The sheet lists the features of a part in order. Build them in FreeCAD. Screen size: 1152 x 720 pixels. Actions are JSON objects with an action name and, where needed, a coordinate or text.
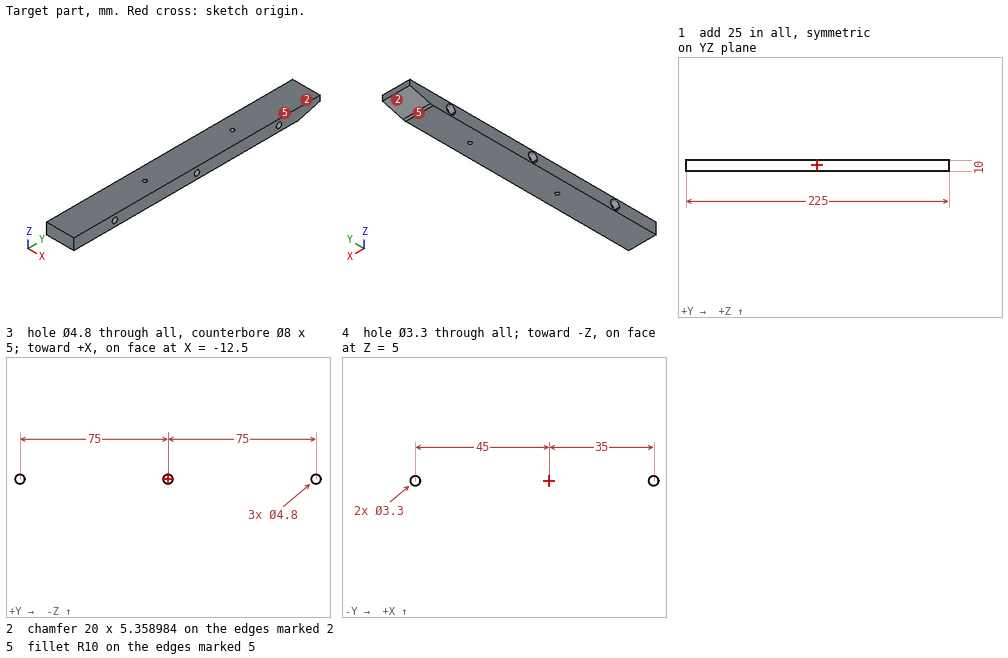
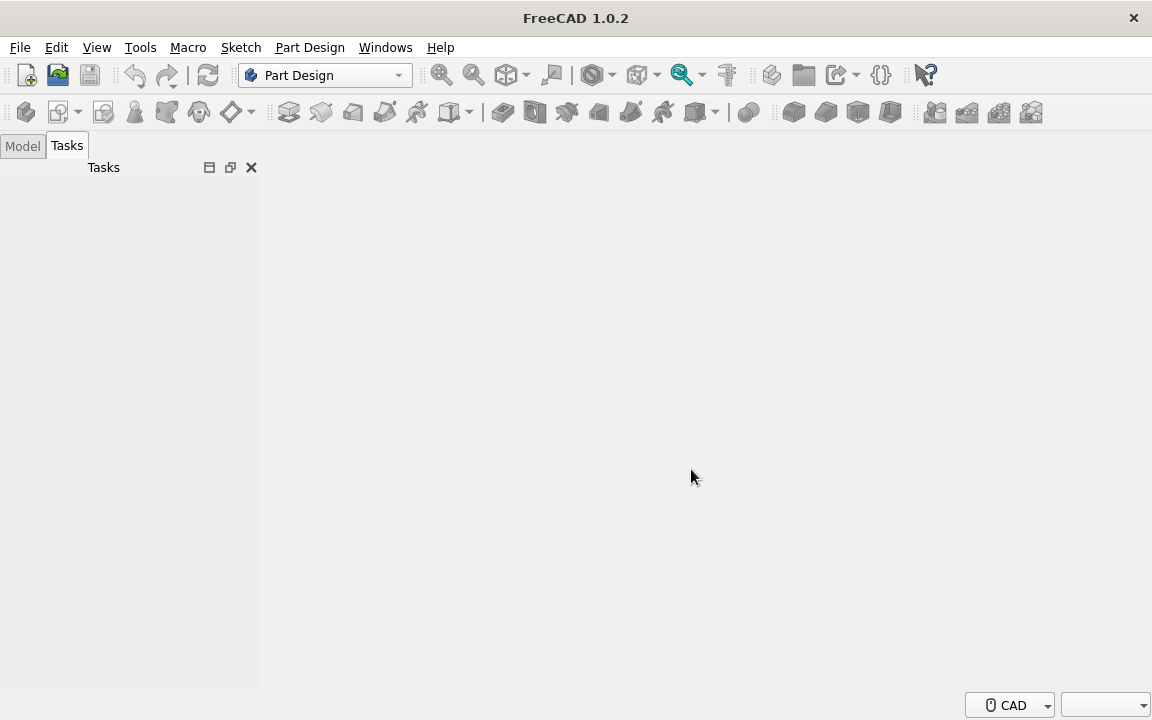
{"action": "key", "text": "ctrl+n"}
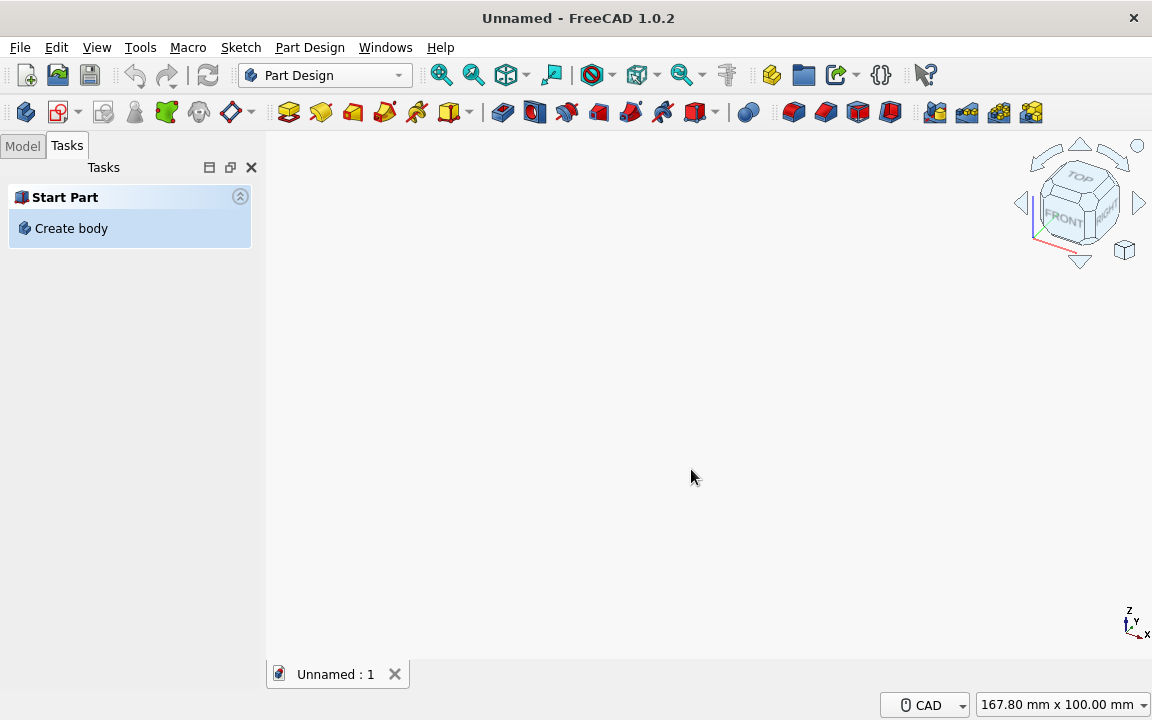
{"action": "left_click", "coordinate": [58, 112]}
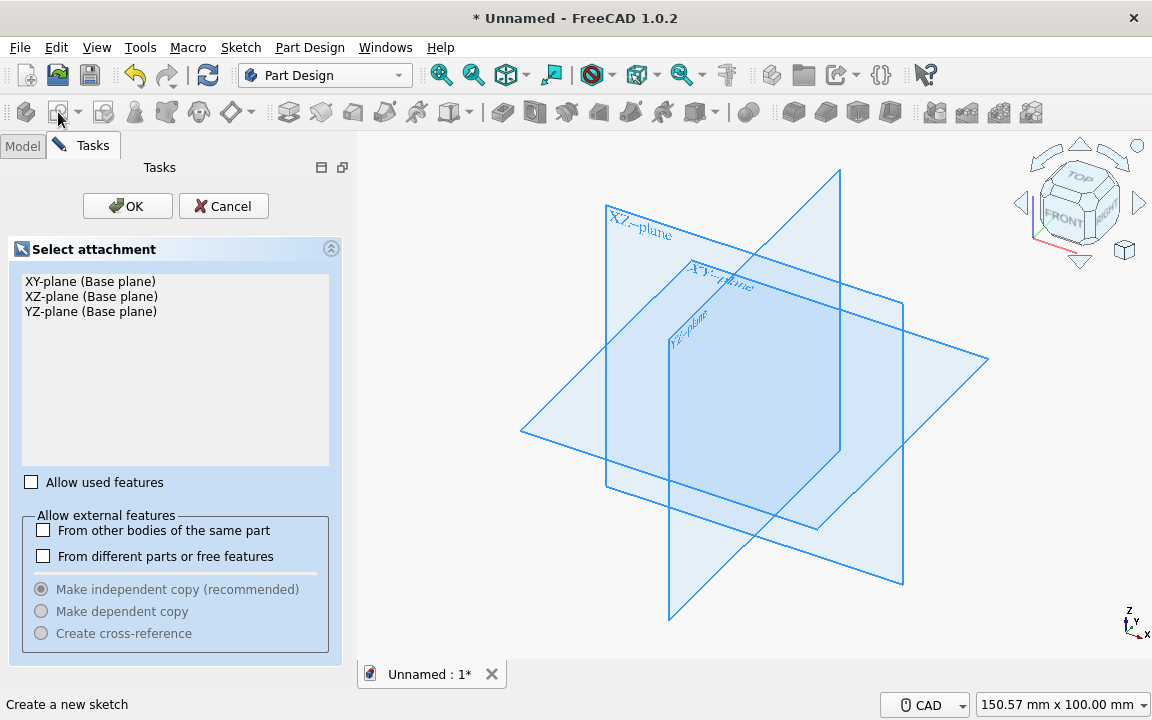
{"action": "left_click", "coordinate": [82, 312]}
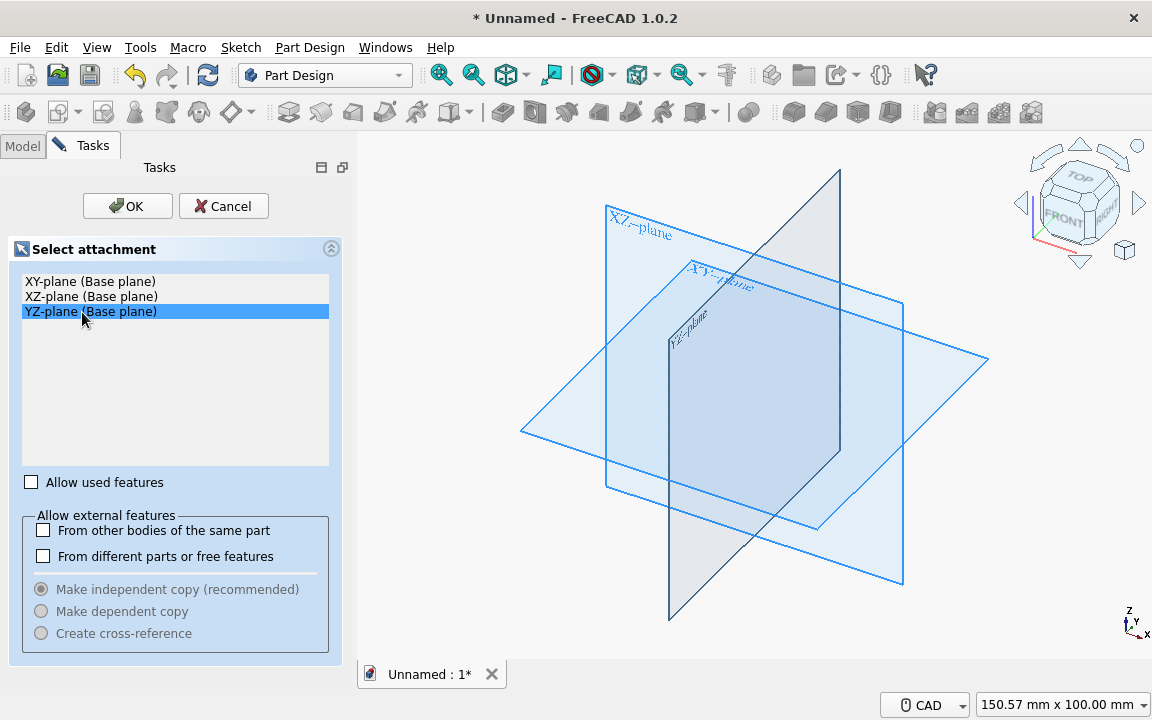
{"action": "left_click", "coordinate": [128, 206]}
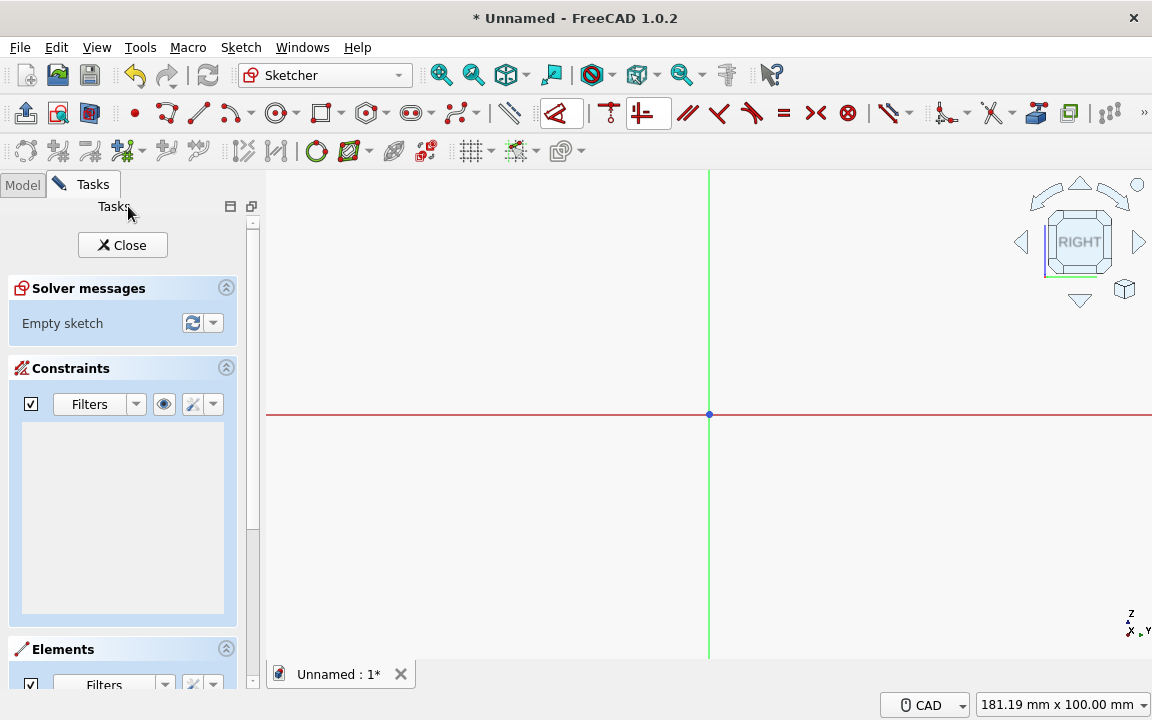
{"action": "scroll", "coordinate": [585, 414], "scroll_direction": "down", "scroll_amount": 4}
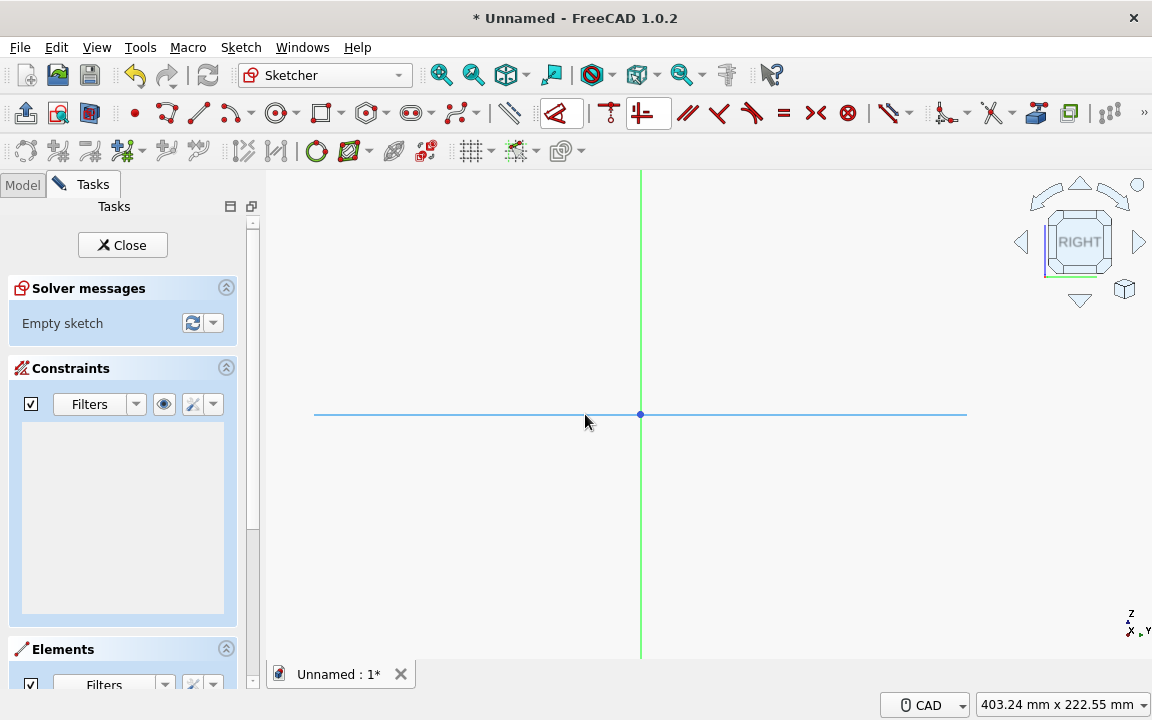
{"action": "left_click", "coordinate": [344, 114]}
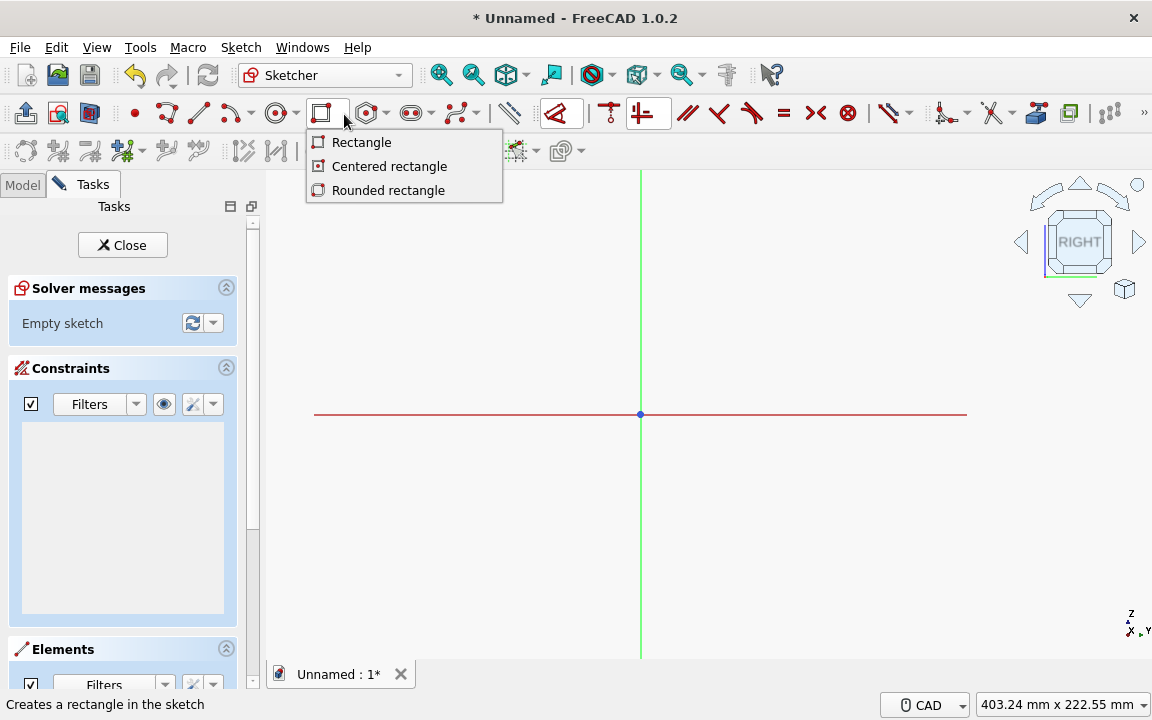
{"action": "left_click", "coordinate": [404, 166]}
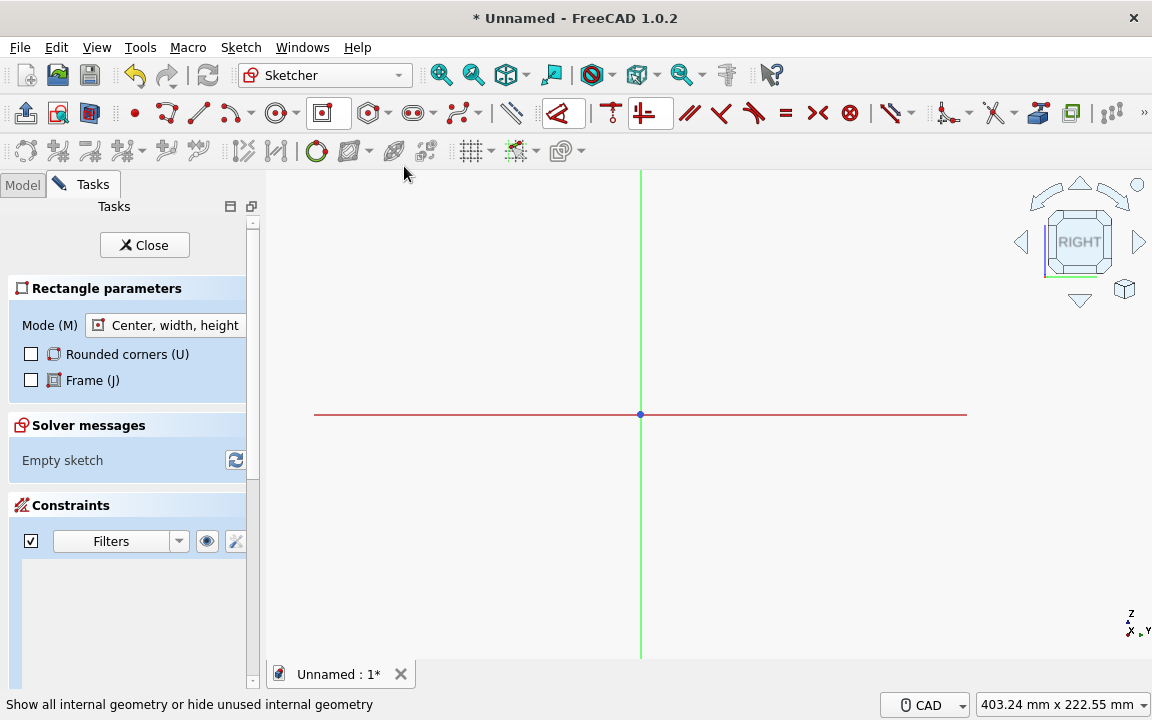
{"action": "scroll", "coordinate": [641, 414], "scroll_direction": "up", "scroll_amount": 2}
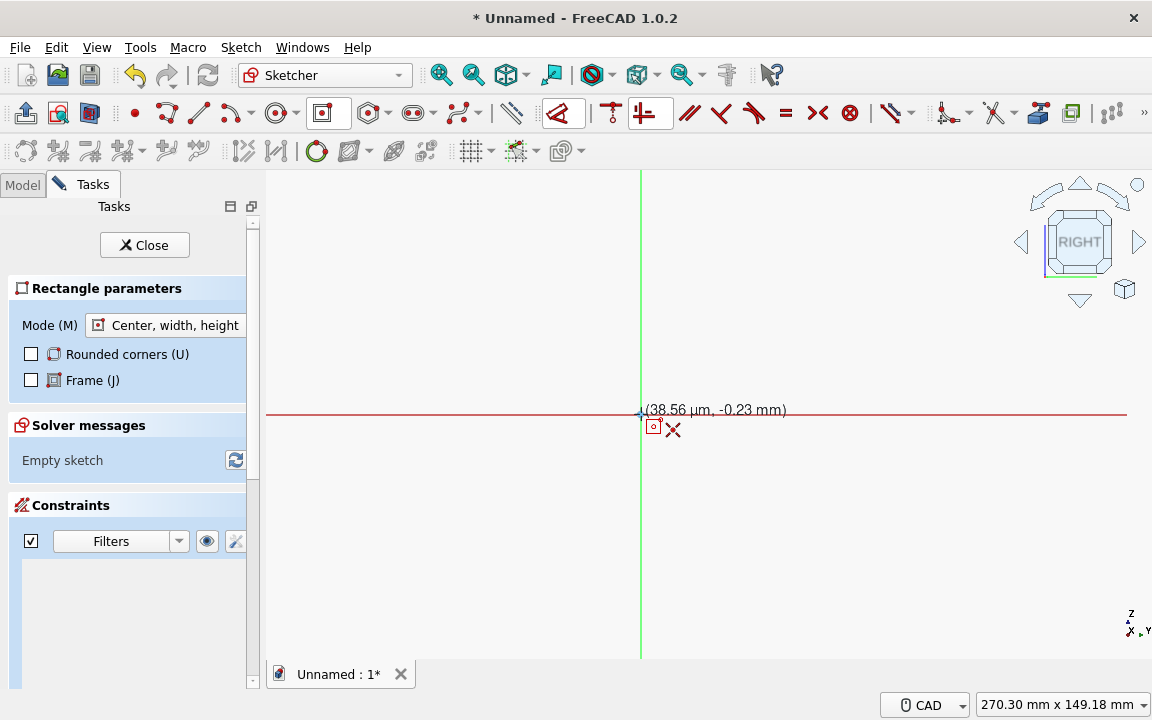
{"action": "left_click", "coordinate": [641, 414]}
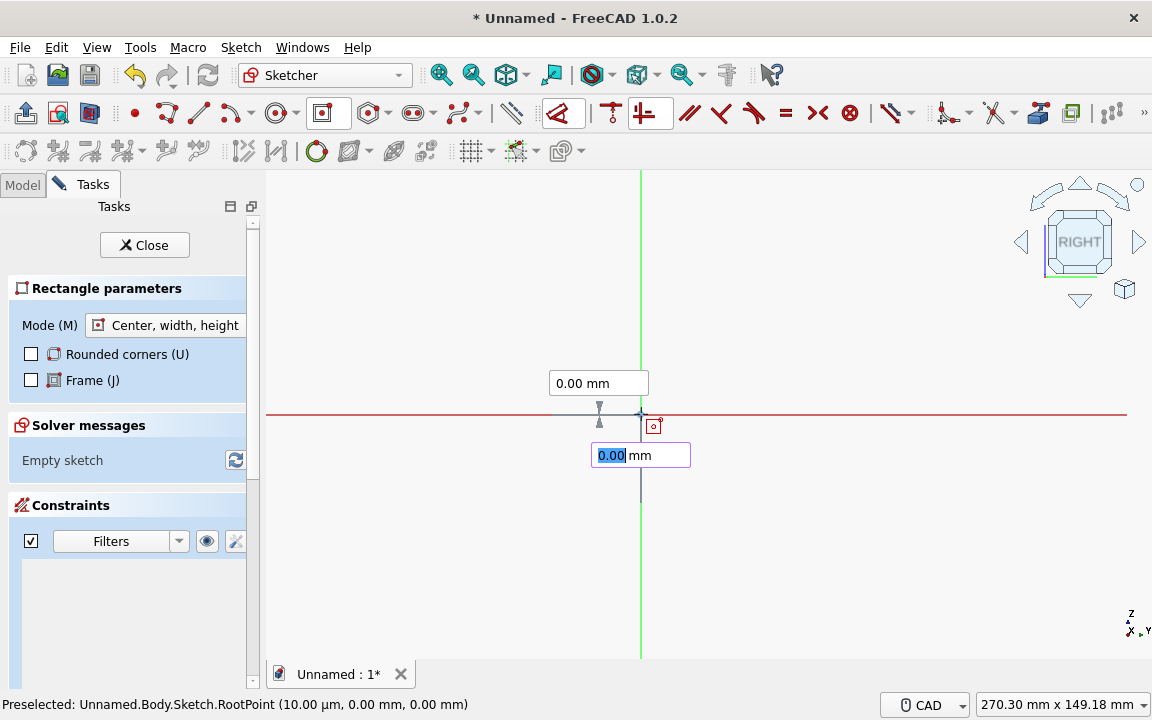
{"action": "scroll", "coordinate": [640, 414], "scroll_direction": "down", "scroll_amount": 2}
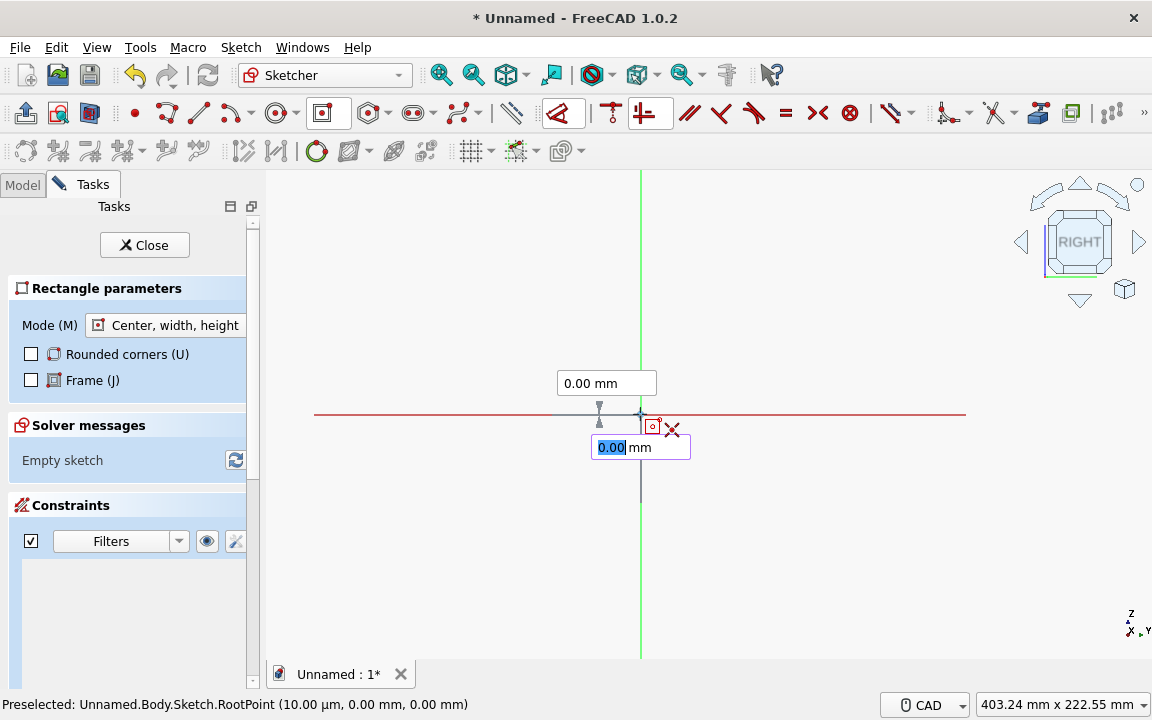
{"action": "scroll", "coordinate": [888, 404], "scroll_direction": "up", "scroll_amount": 2}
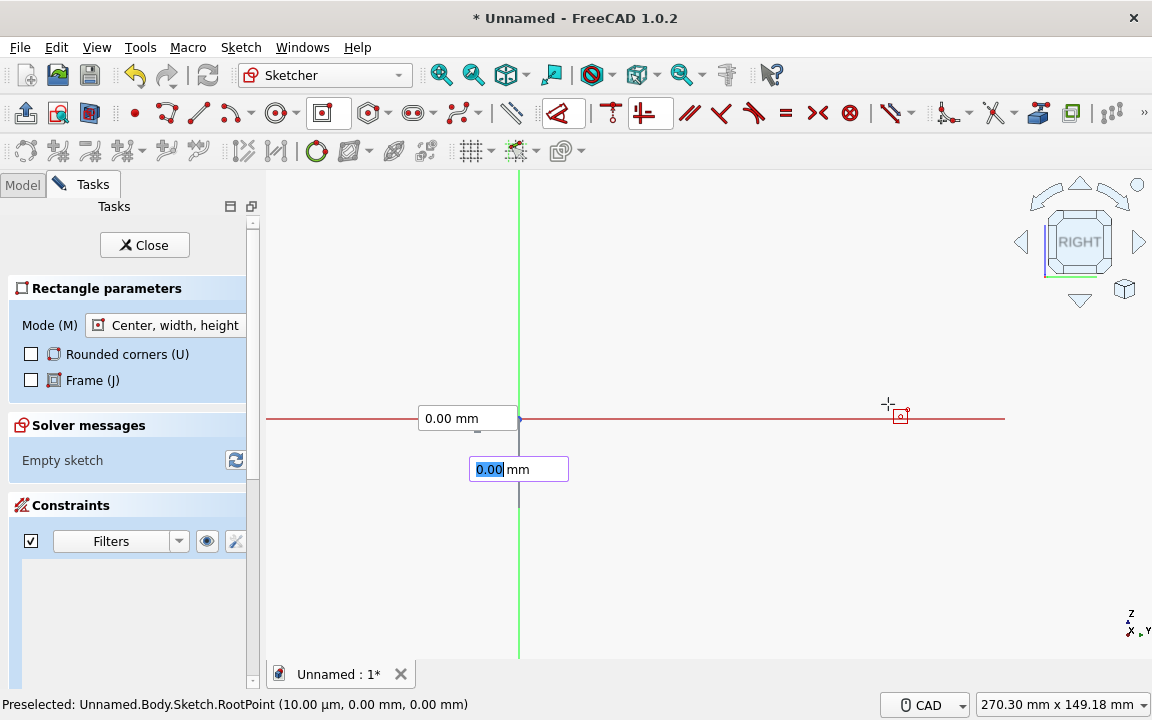
{"action": "left_click", "coordinate": [887, 403]}
{"action": "key", "text": "Escape"}